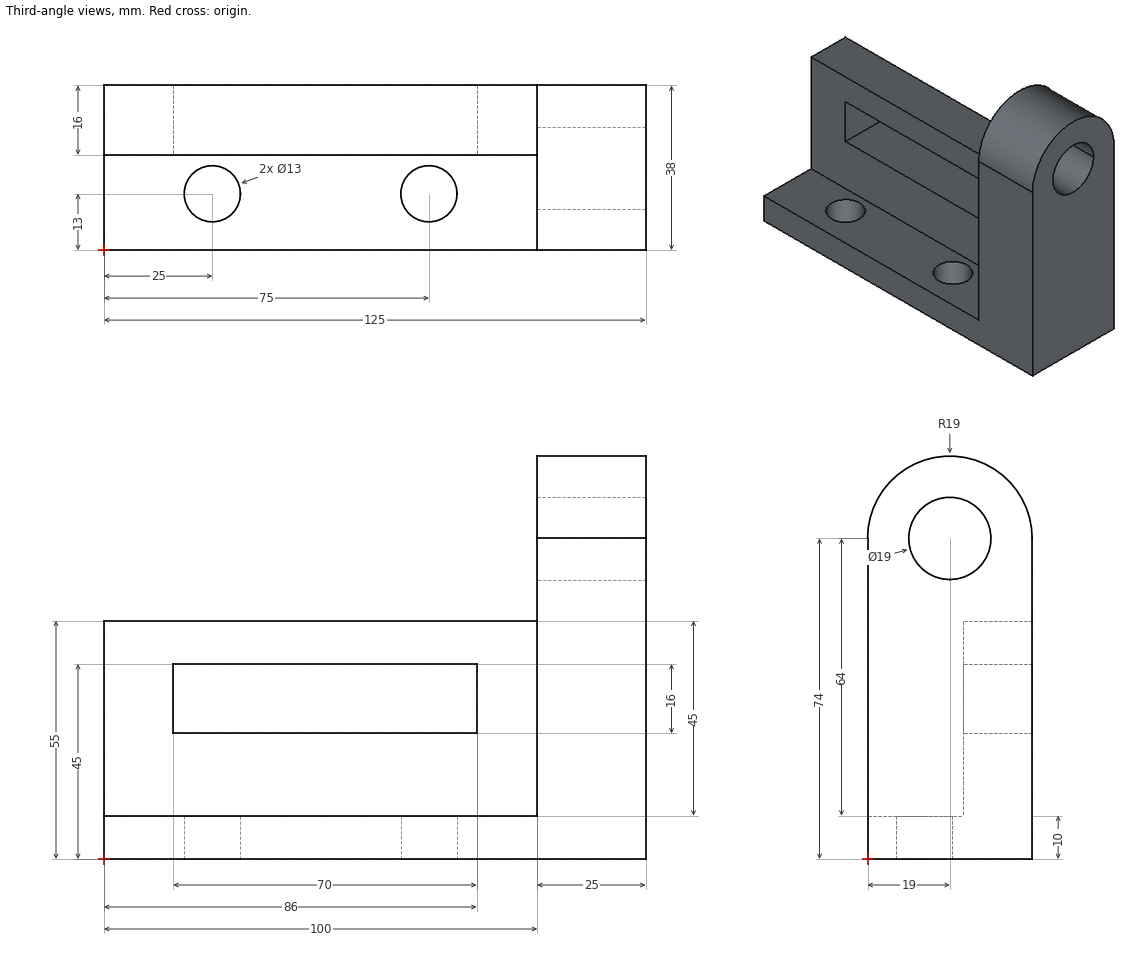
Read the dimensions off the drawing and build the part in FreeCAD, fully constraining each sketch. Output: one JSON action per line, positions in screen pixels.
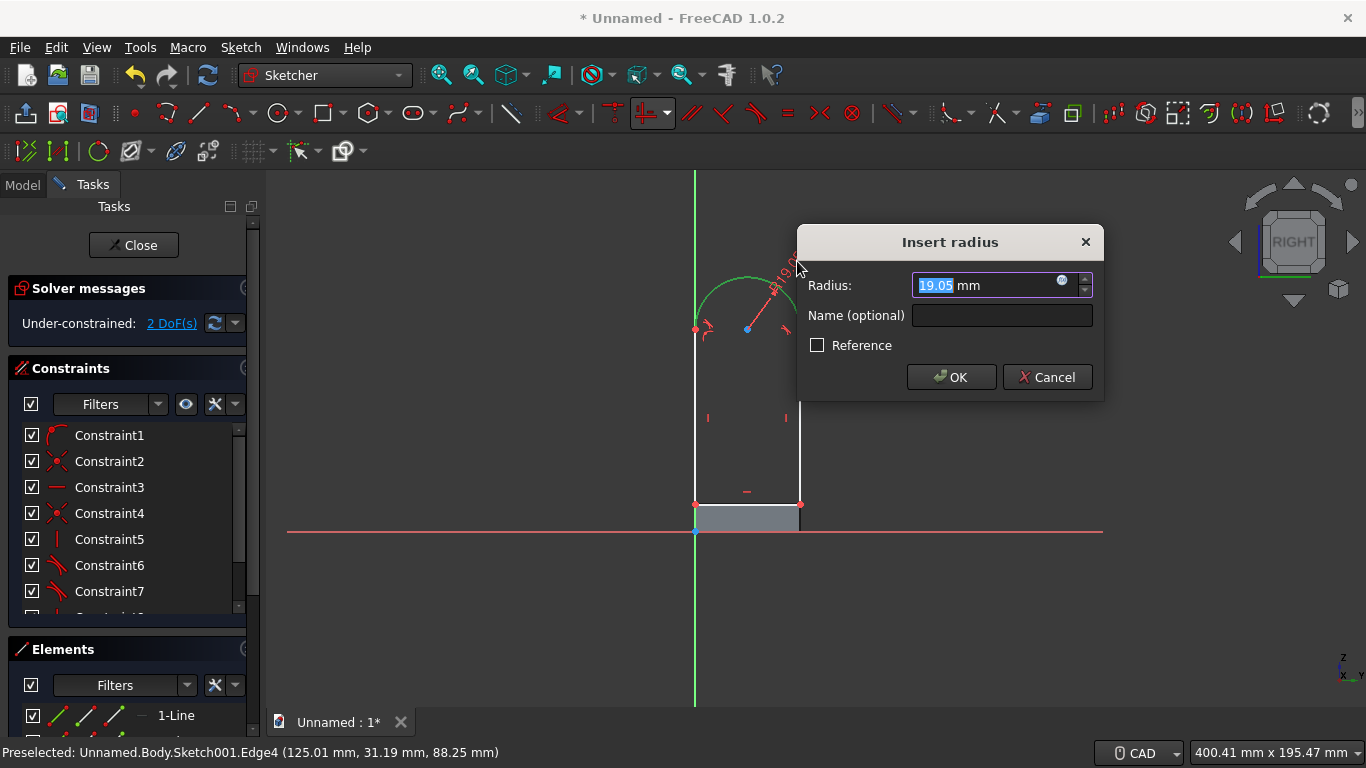
{"action": "type", "text": "19"}
{"action": "key", "text": "Return"}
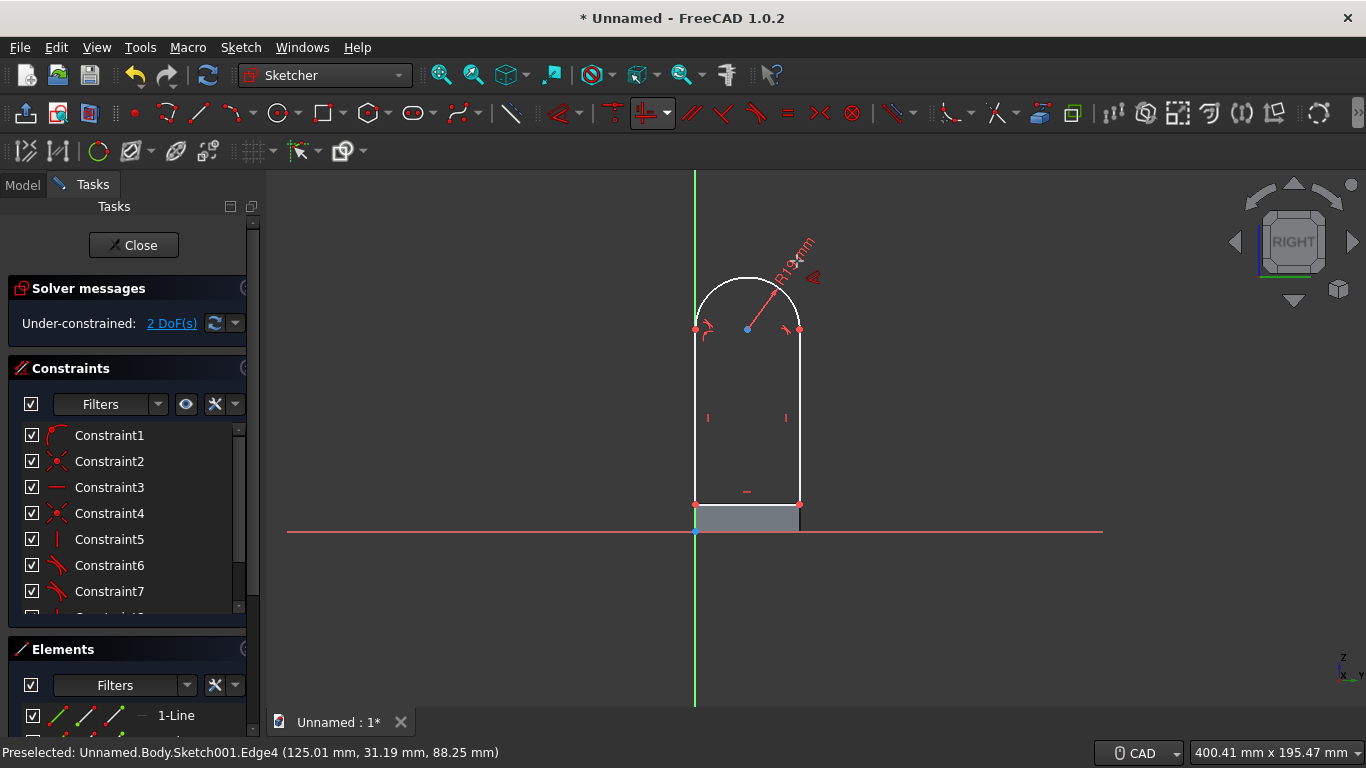
{"action": "left_click", "coordinate": [695, 382]}
{"action": "left_click", "coordinate": [661, 417]}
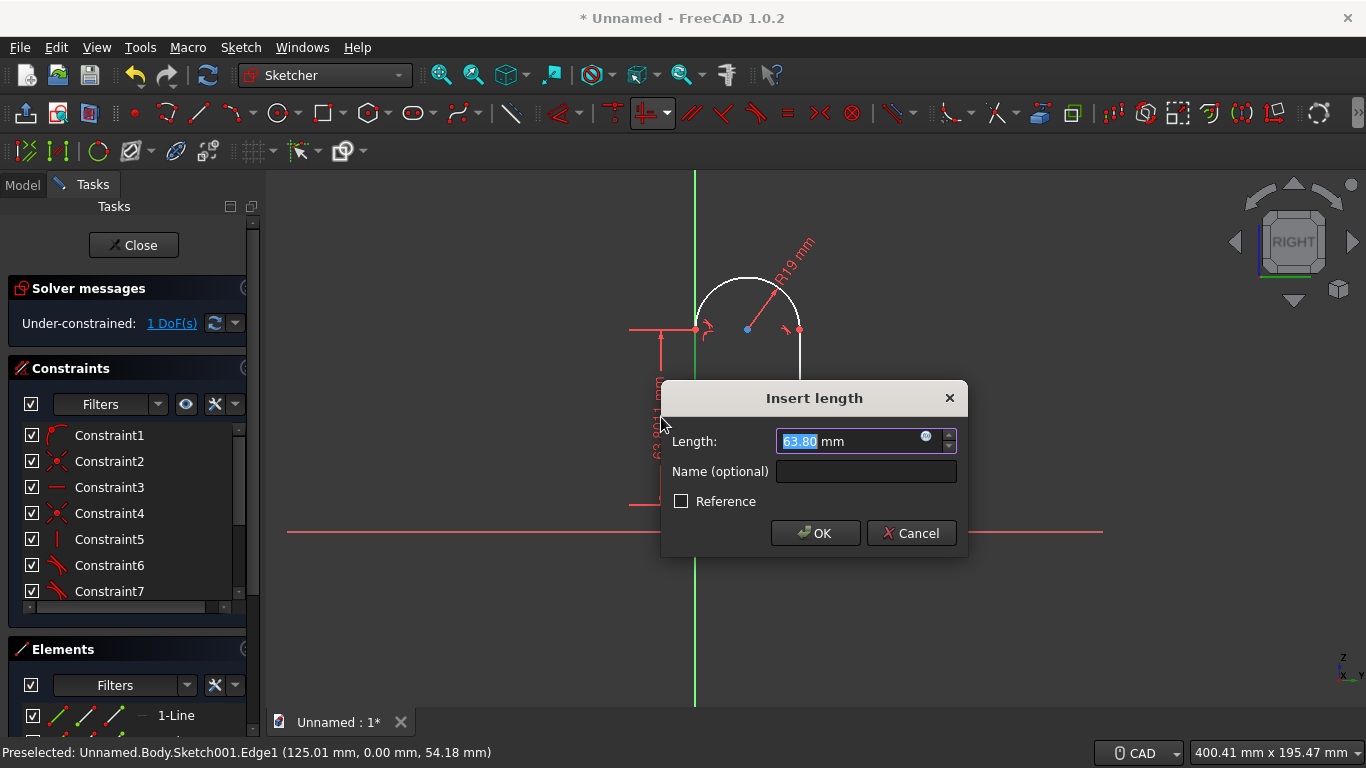
{"action": "type", "text": "64"}
{"action": "key", "text": "Return"}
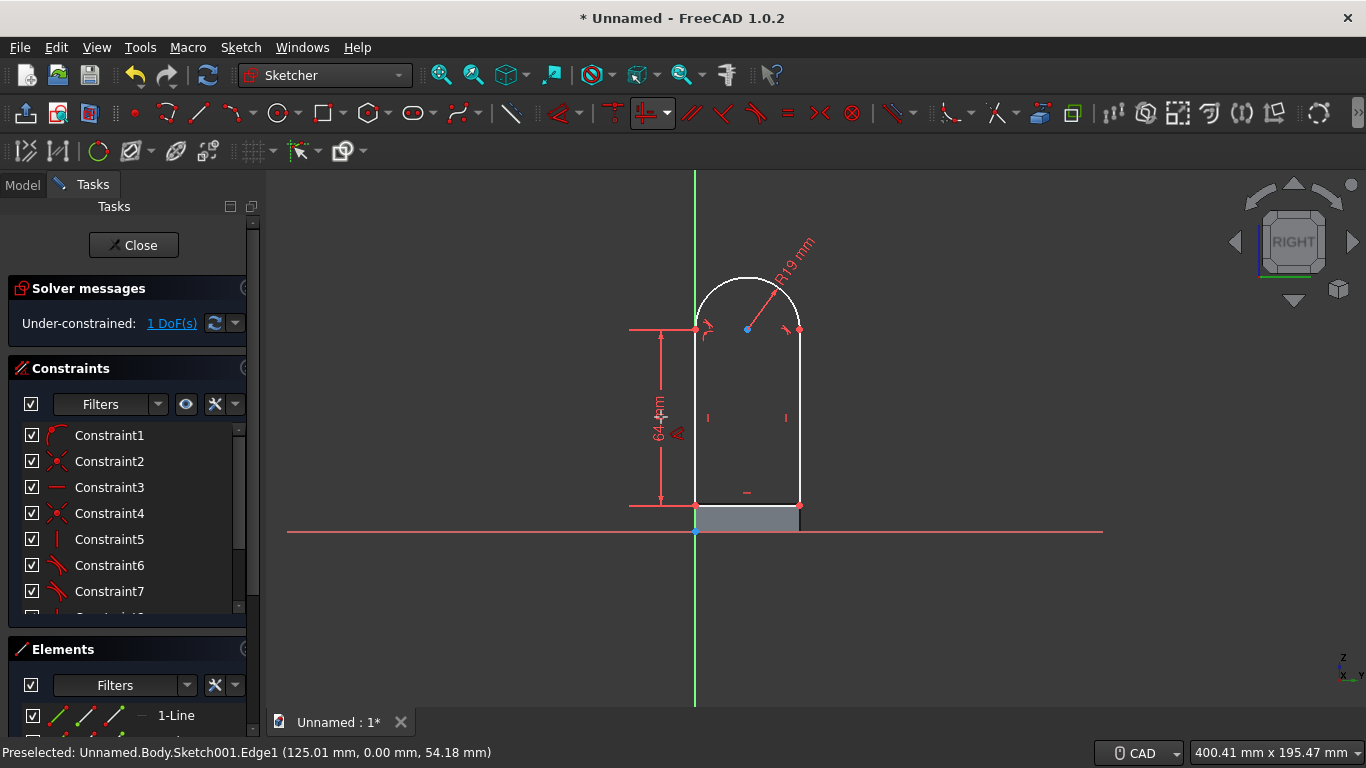
{"action": "left_click", "coordinate": [695, 330]}
{"action": "left_click", "coordinate": [661, 384]}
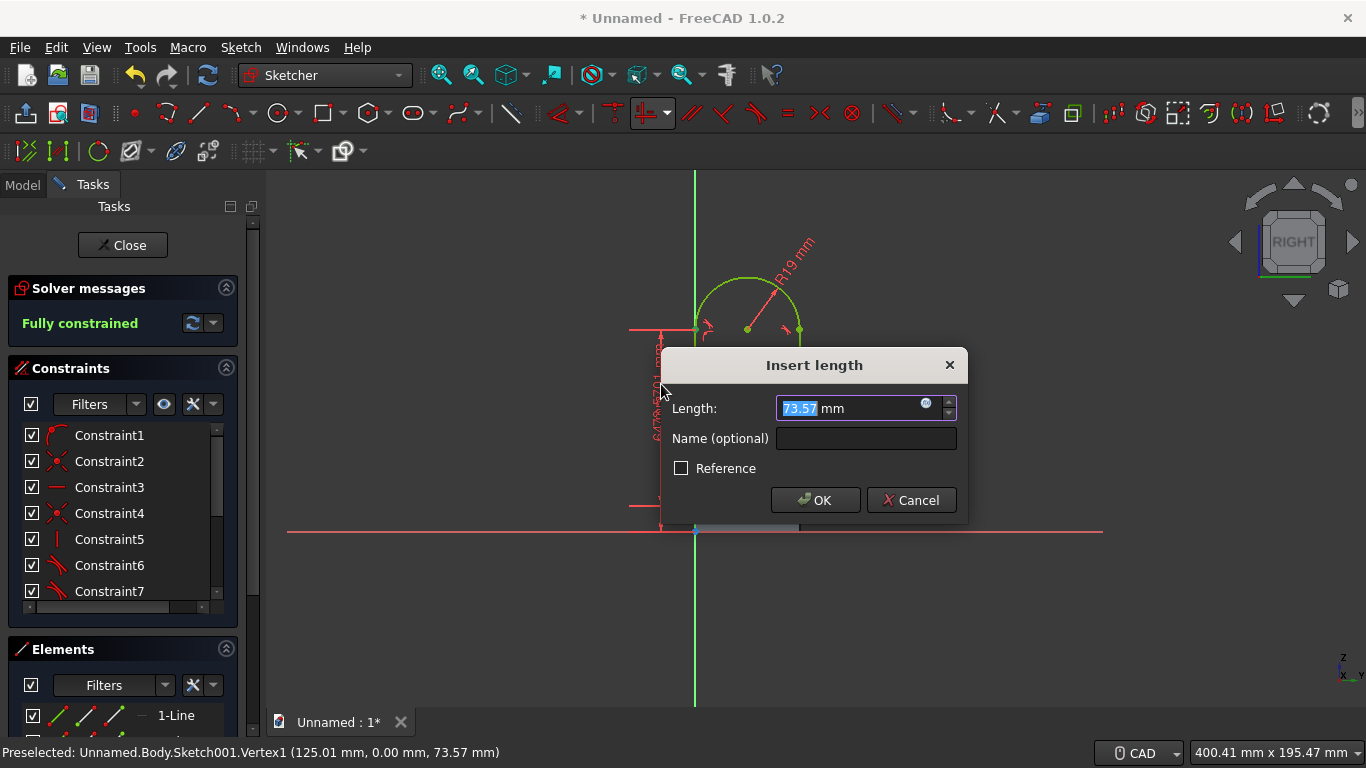
{"action": "type", "text": "74"}
{"action": "key", "text": "Return"}
{"action": "key", "text": "Escape"}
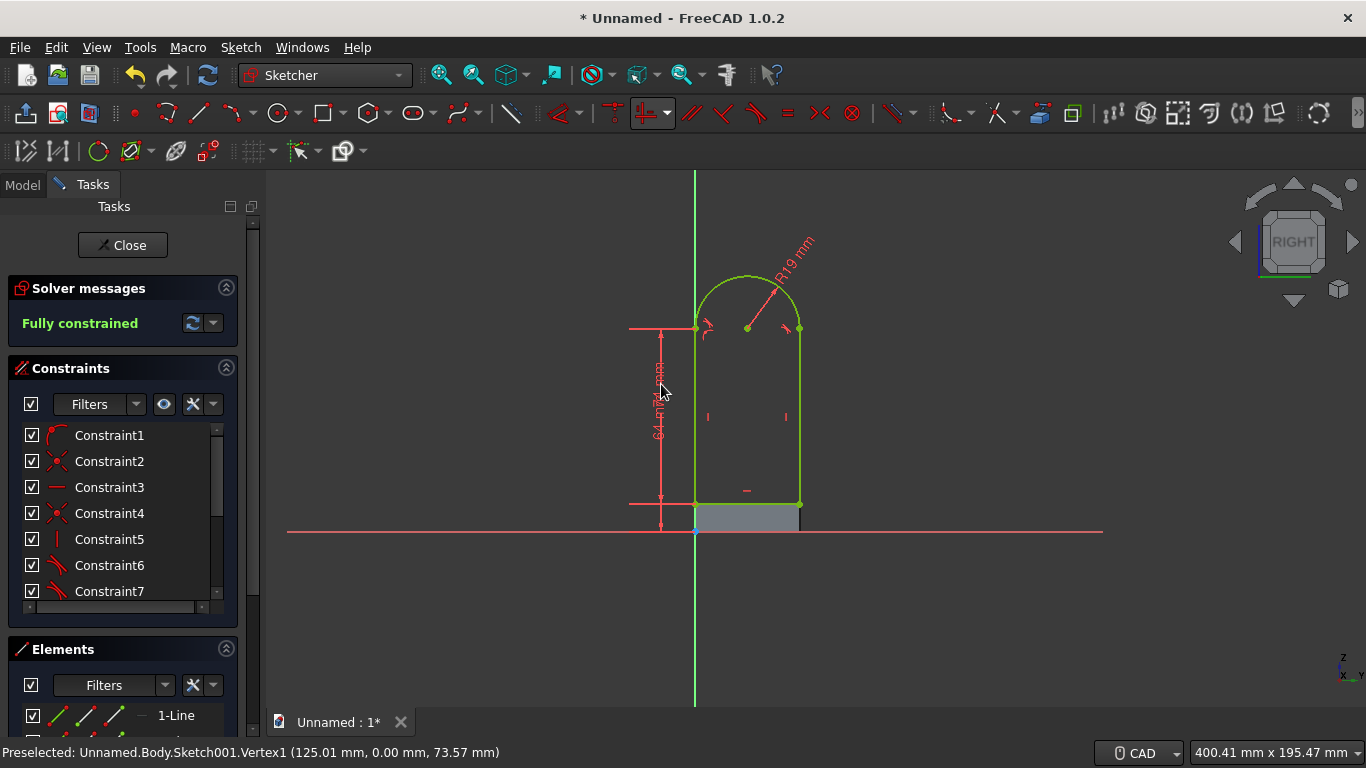
{"action": "left_click", "coordinate": [123, 245]}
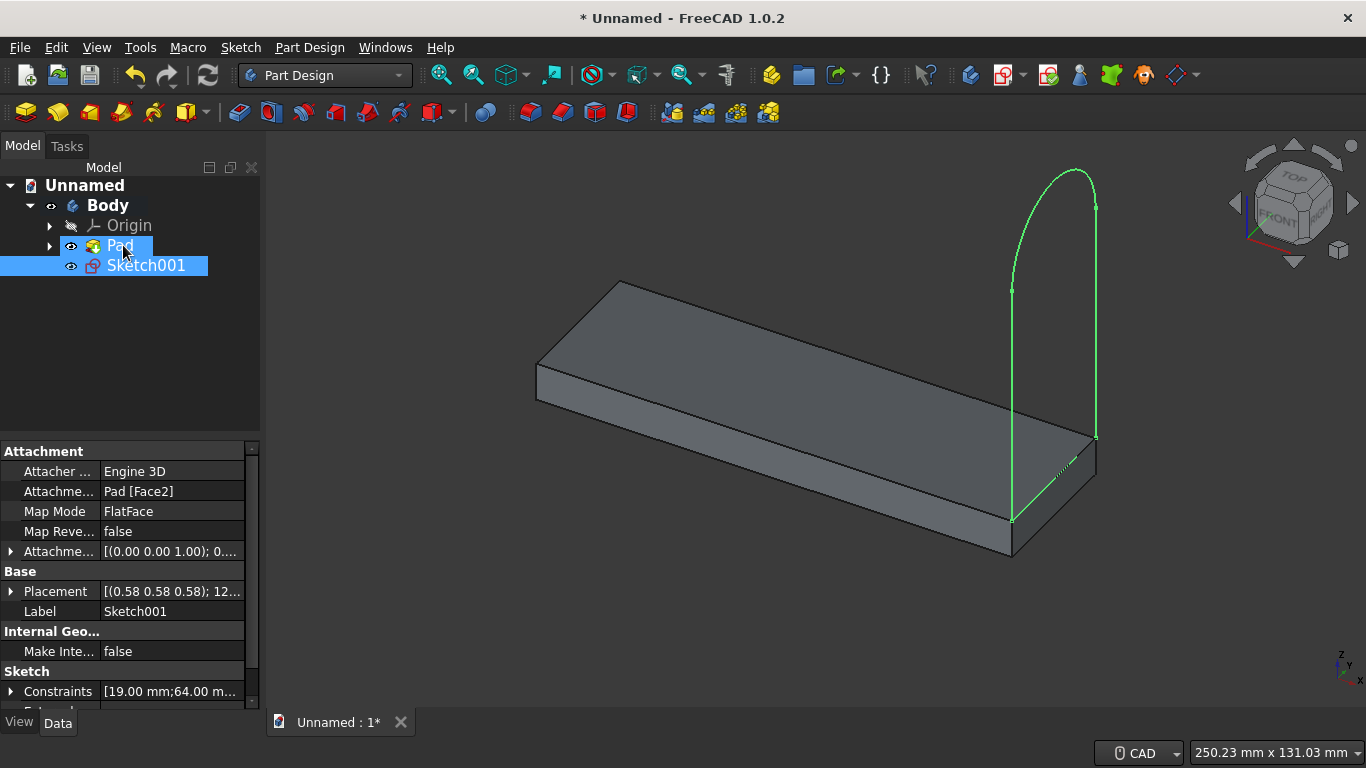
{"action": "left_click", "coordinate": [26, 112]}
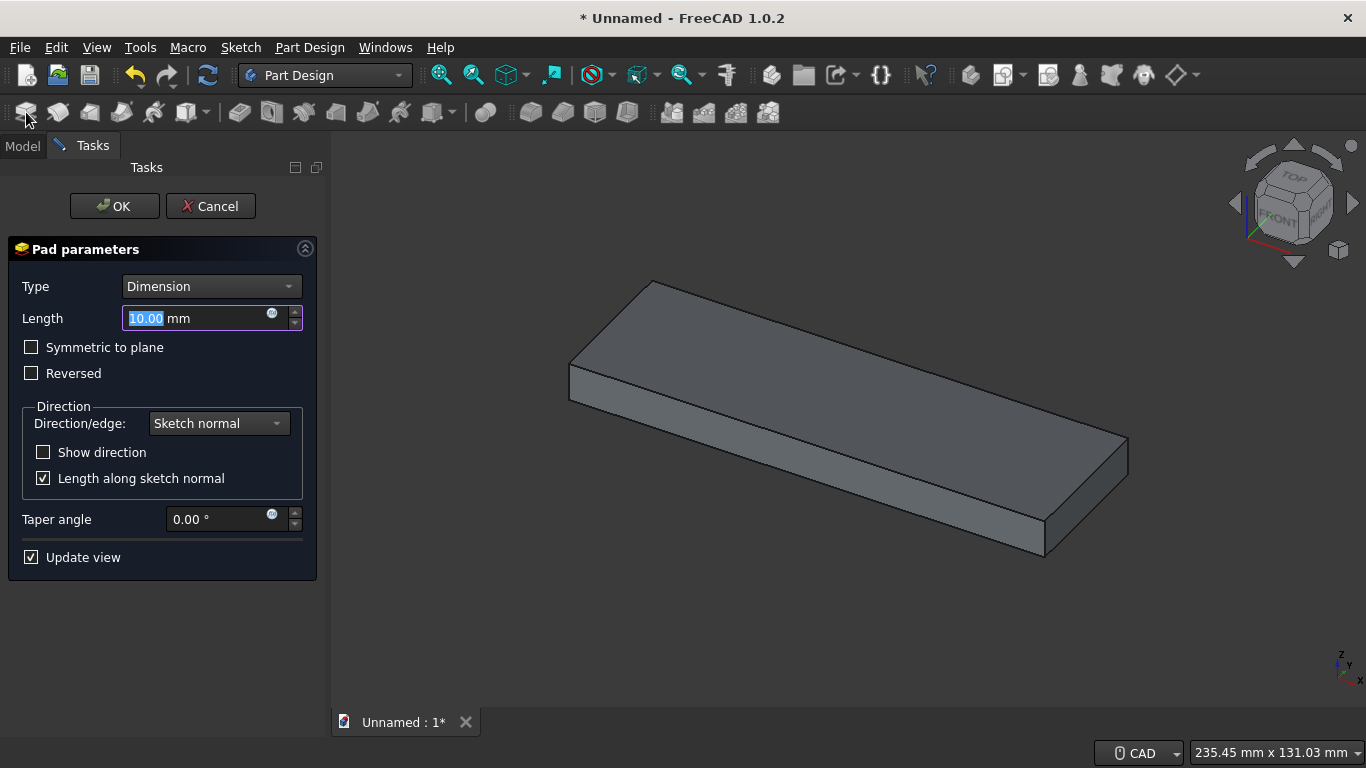
{"action": "type", "text": "25"}
{"action": "key", "text": "Tab"}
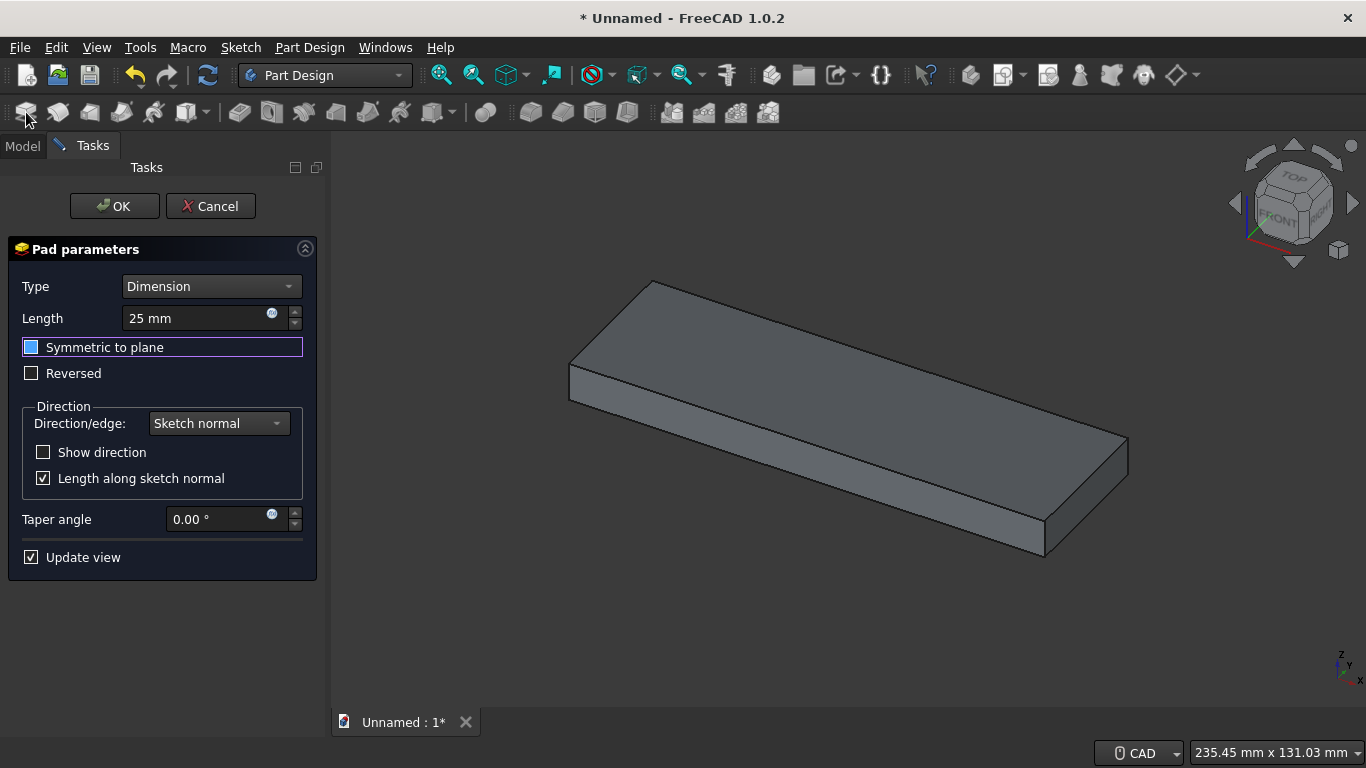
{"action": "left_click", "coordinate": [30, 373]}